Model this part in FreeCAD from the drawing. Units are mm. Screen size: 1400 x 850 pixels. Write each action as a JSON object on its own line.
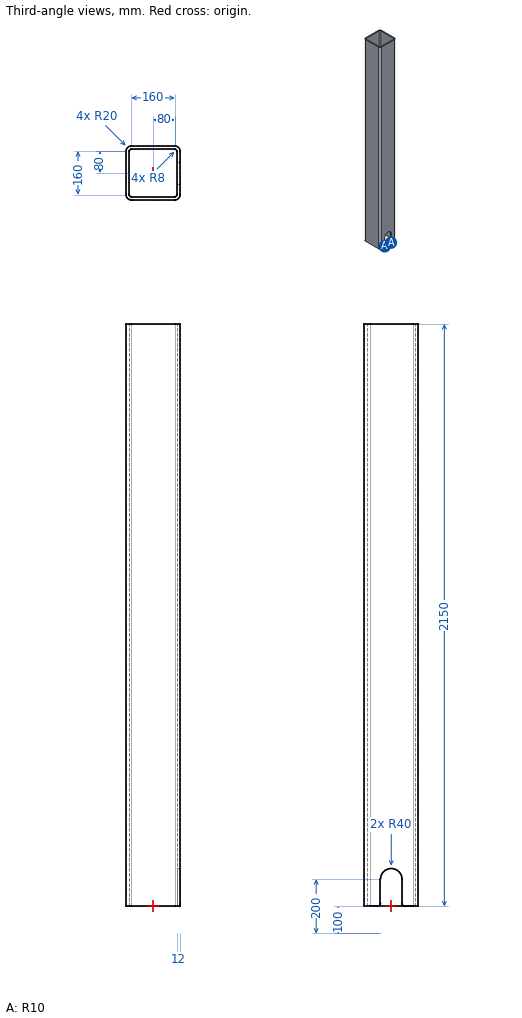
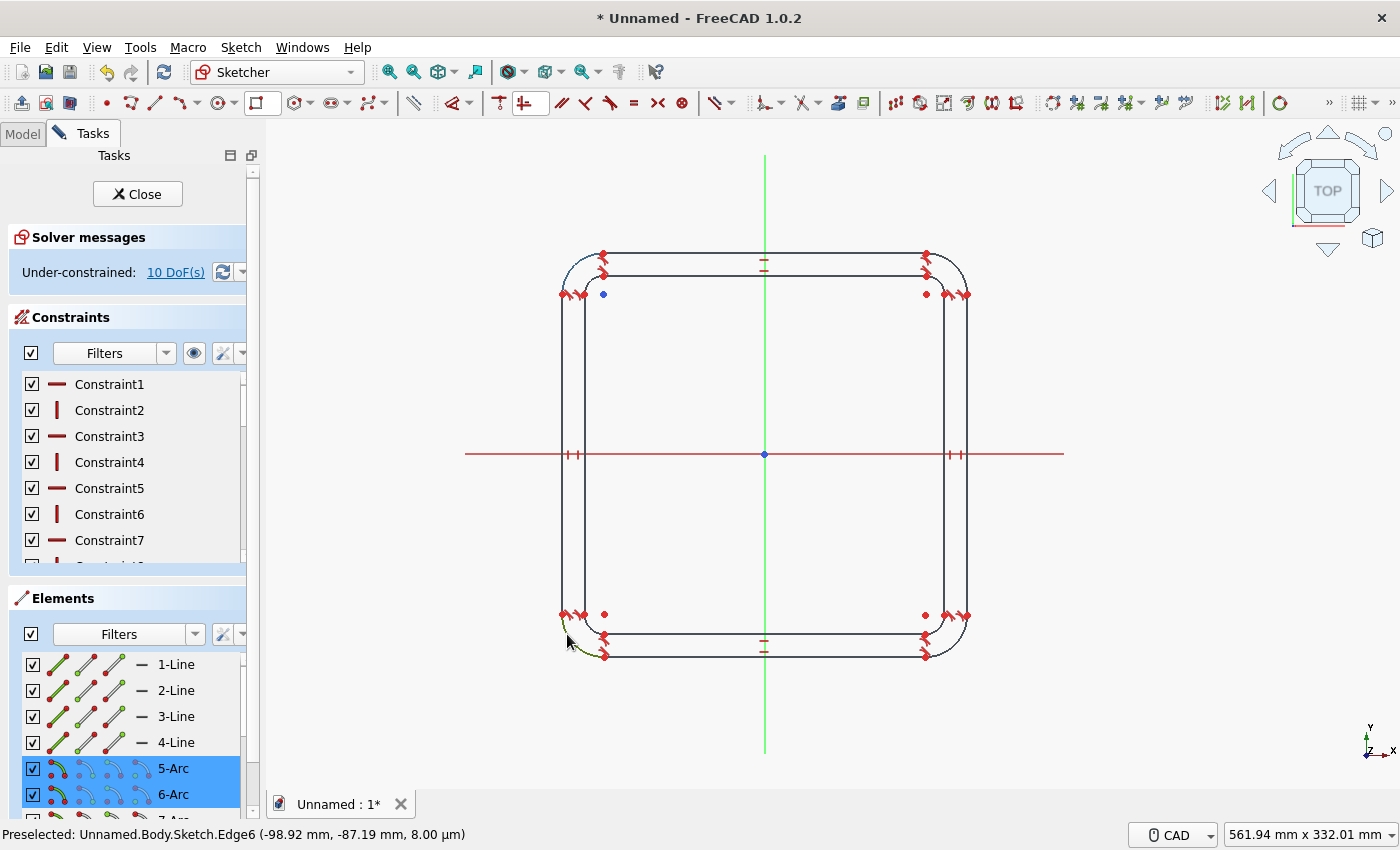
{"action": "left_click", "coordinate": [944, 652]}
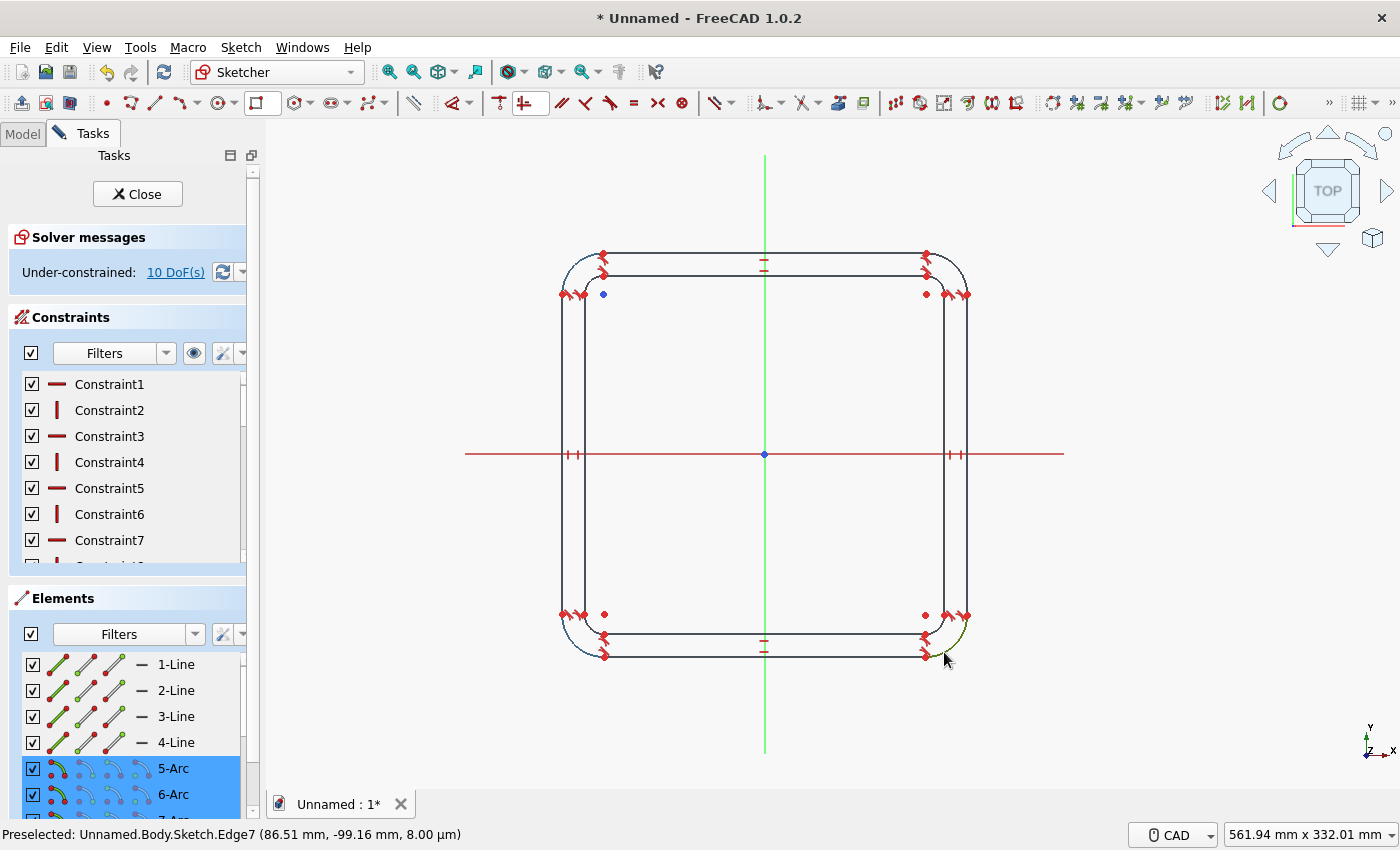
{"action": "left_click", "coordinate": [963, 276]}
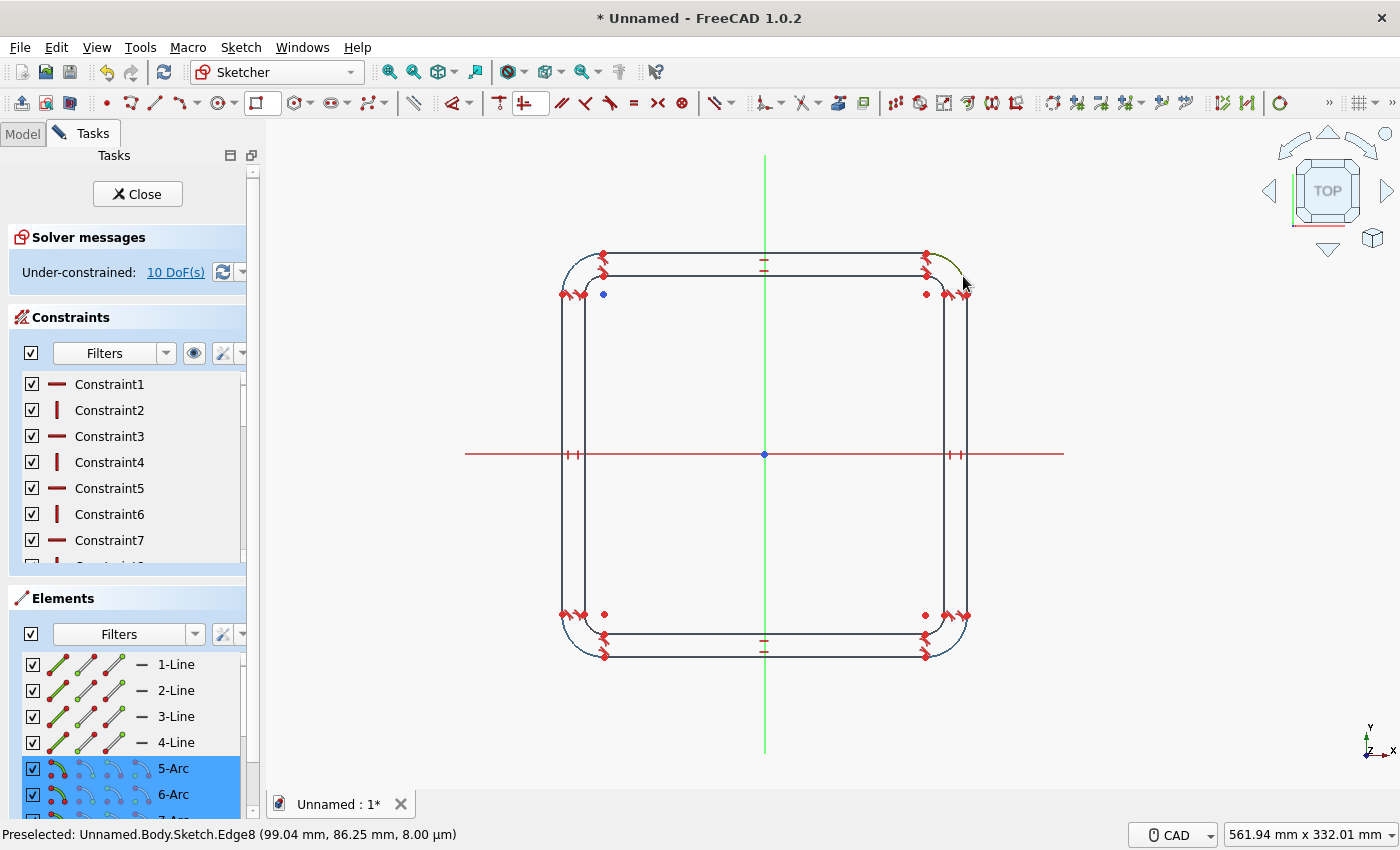
{"action": "left_click", "coordinate": [634, 104]}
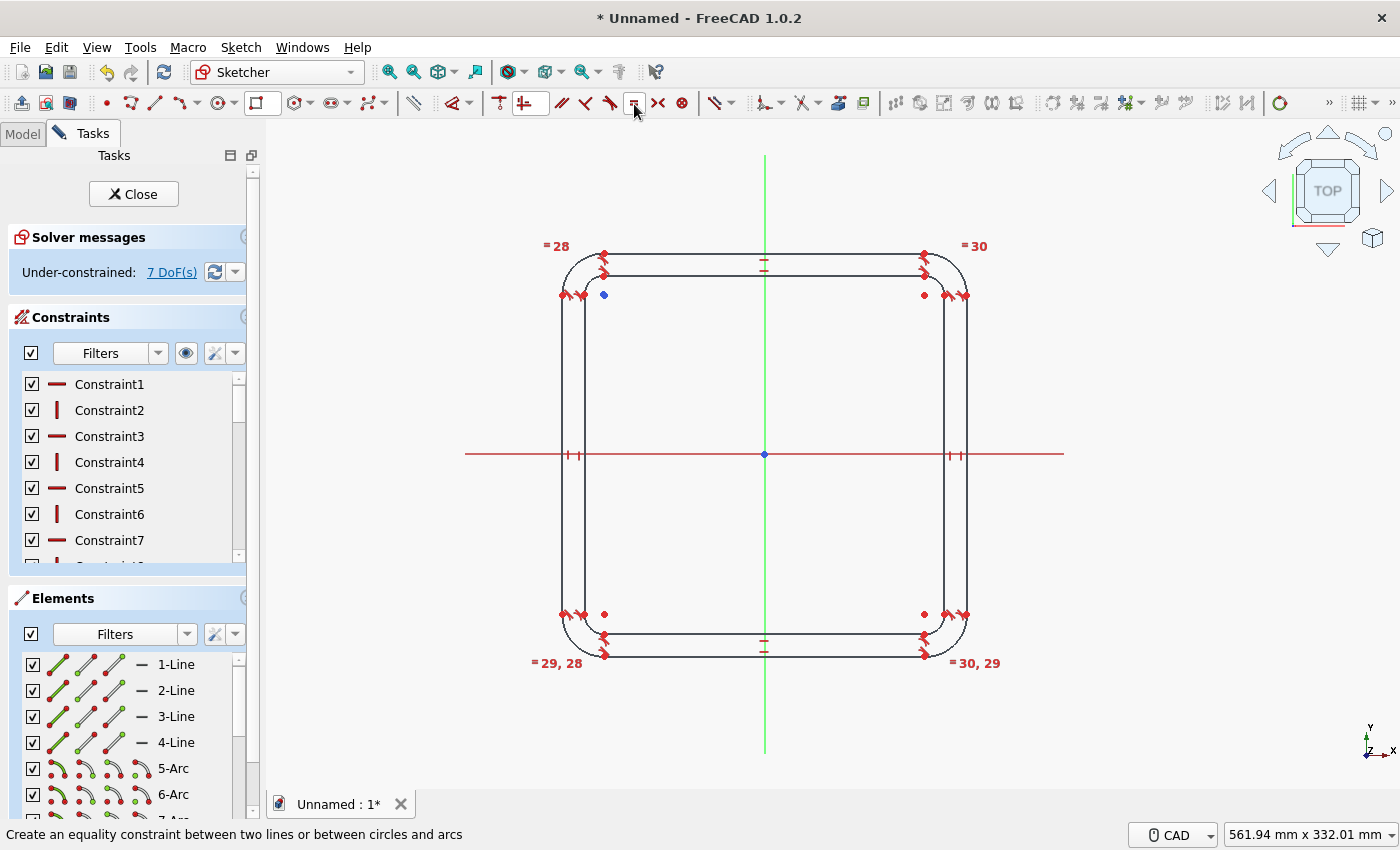
{"action": "scroll", "coordinate": [942, 287], "scroll_direction": "up", "scroll_amount": 3}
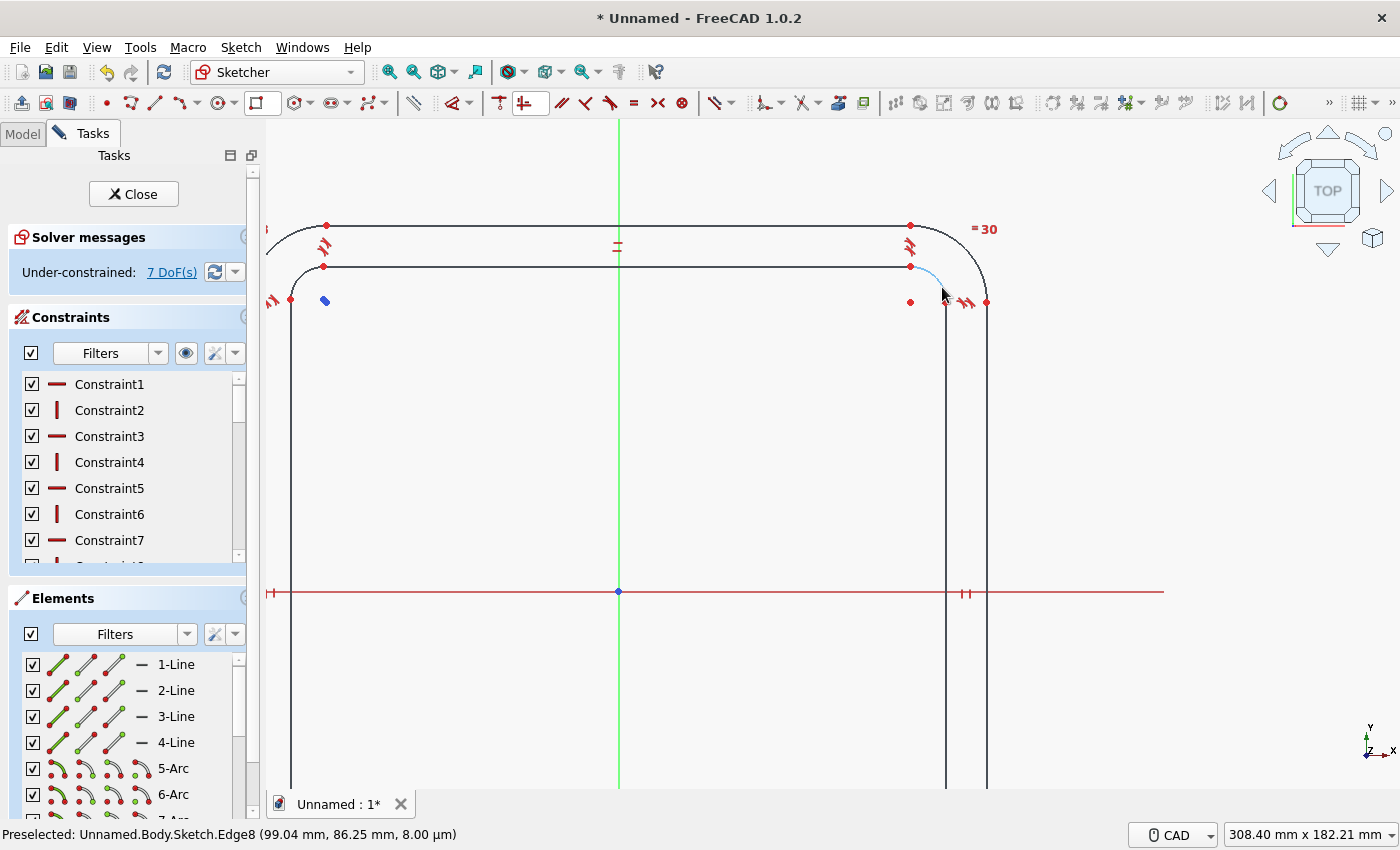
{"action": "left_click", "coordinate": [942, 286]}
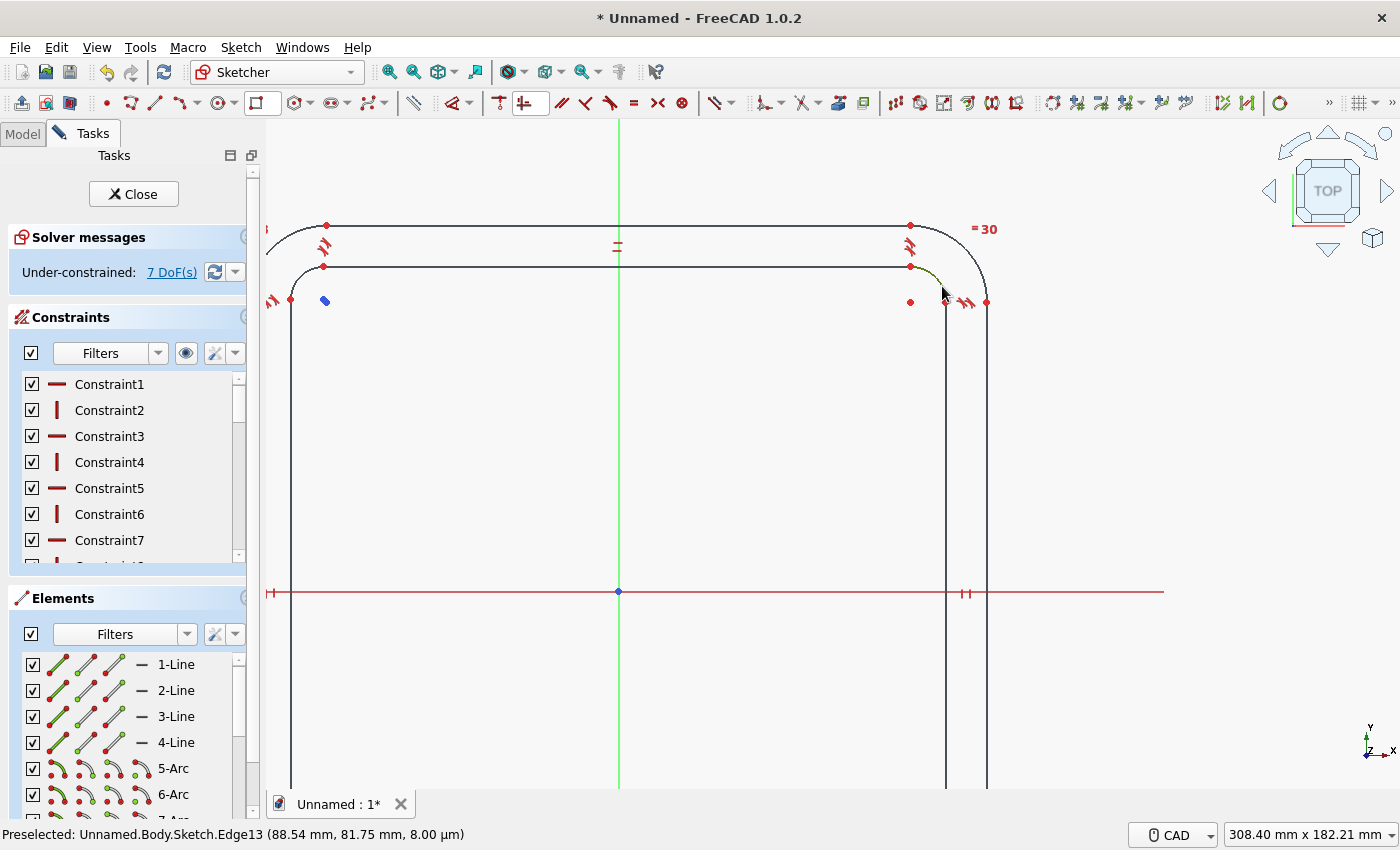
{"action": "left_click", "coordinate": [309, 270]}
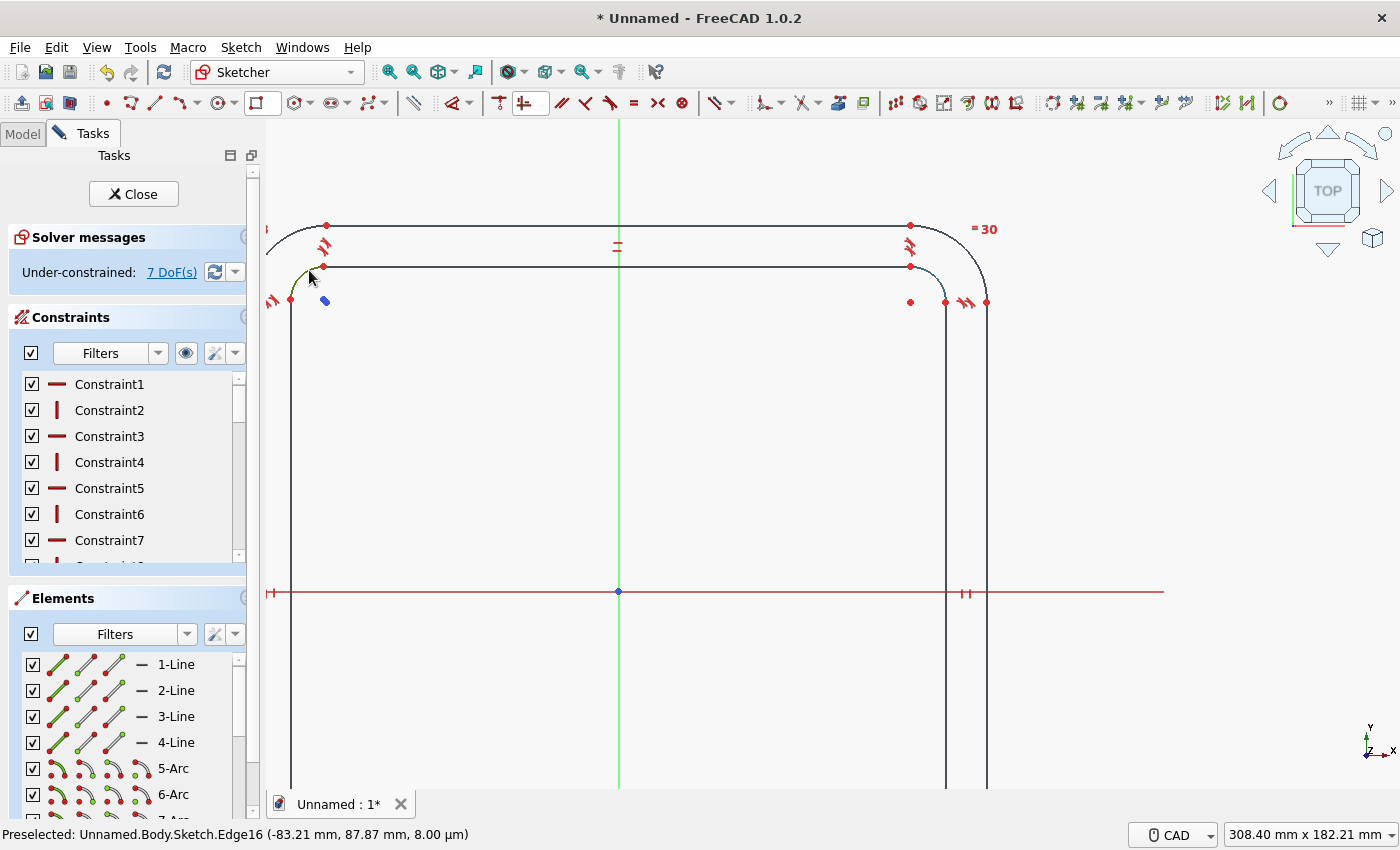
{"action": "left_click", "coordinate": [634, 104]}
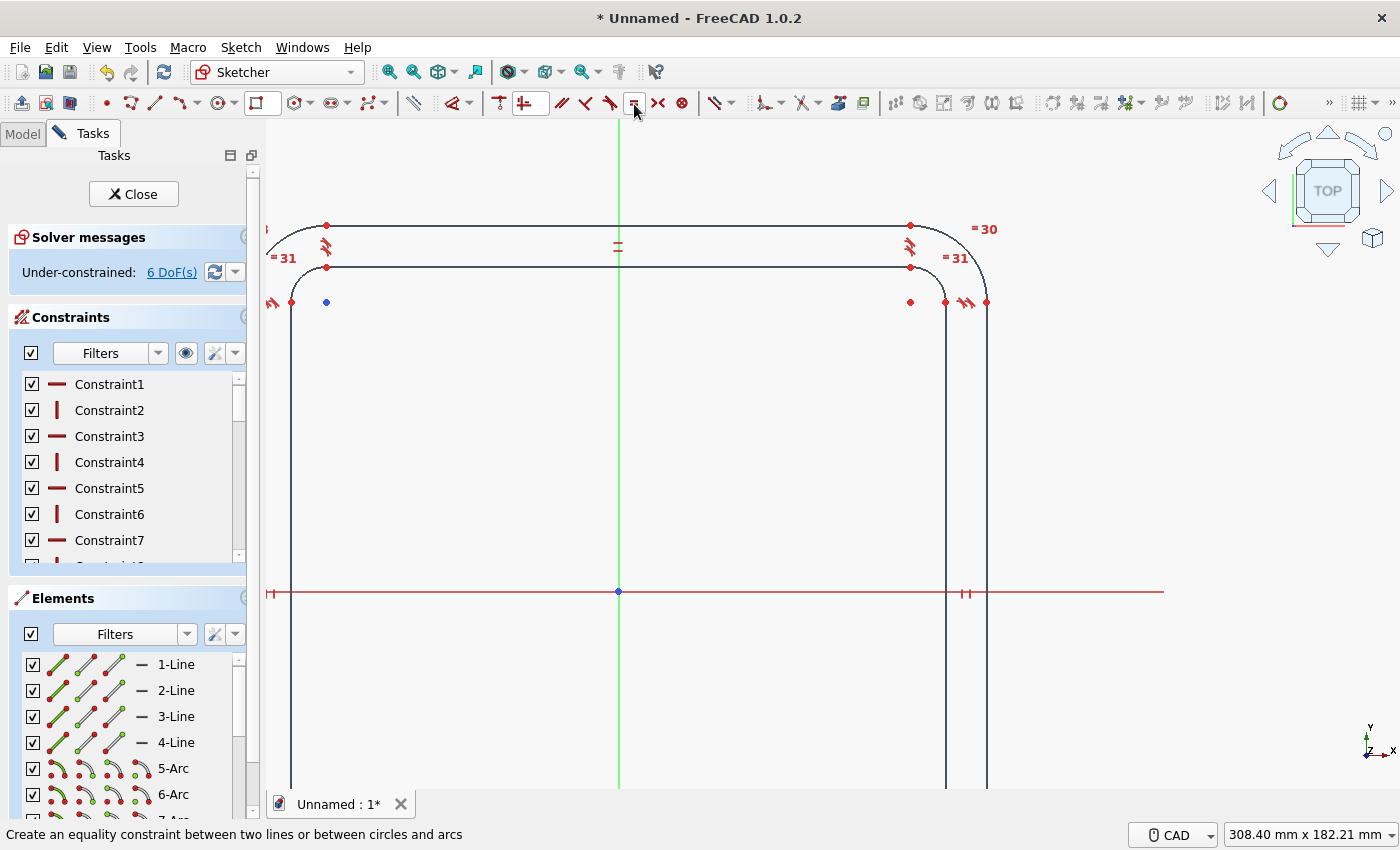
{"action": "left_click", "coordinate": [303, 230]}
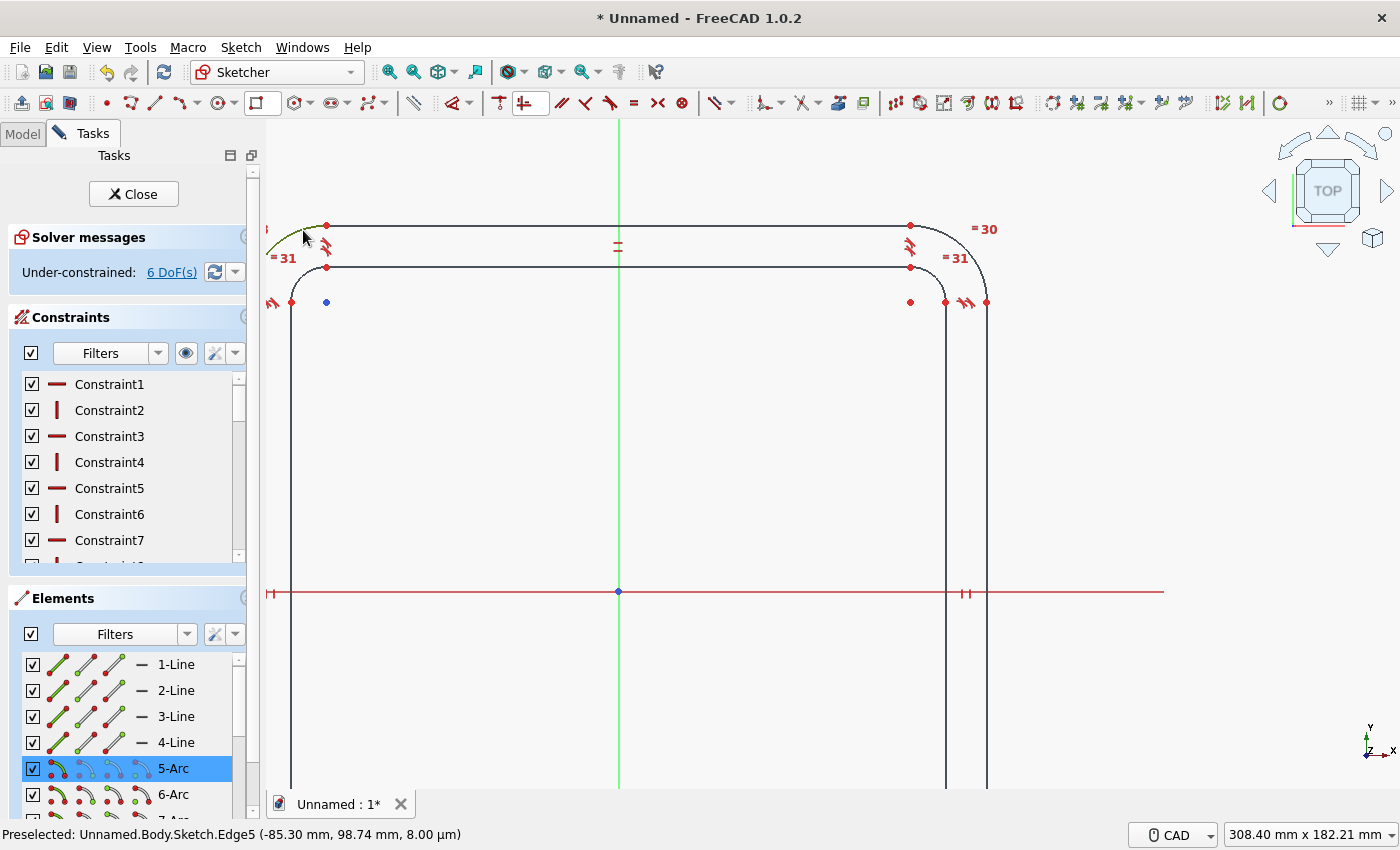
{"action": "left_click", "coordinate": [472, 104]}